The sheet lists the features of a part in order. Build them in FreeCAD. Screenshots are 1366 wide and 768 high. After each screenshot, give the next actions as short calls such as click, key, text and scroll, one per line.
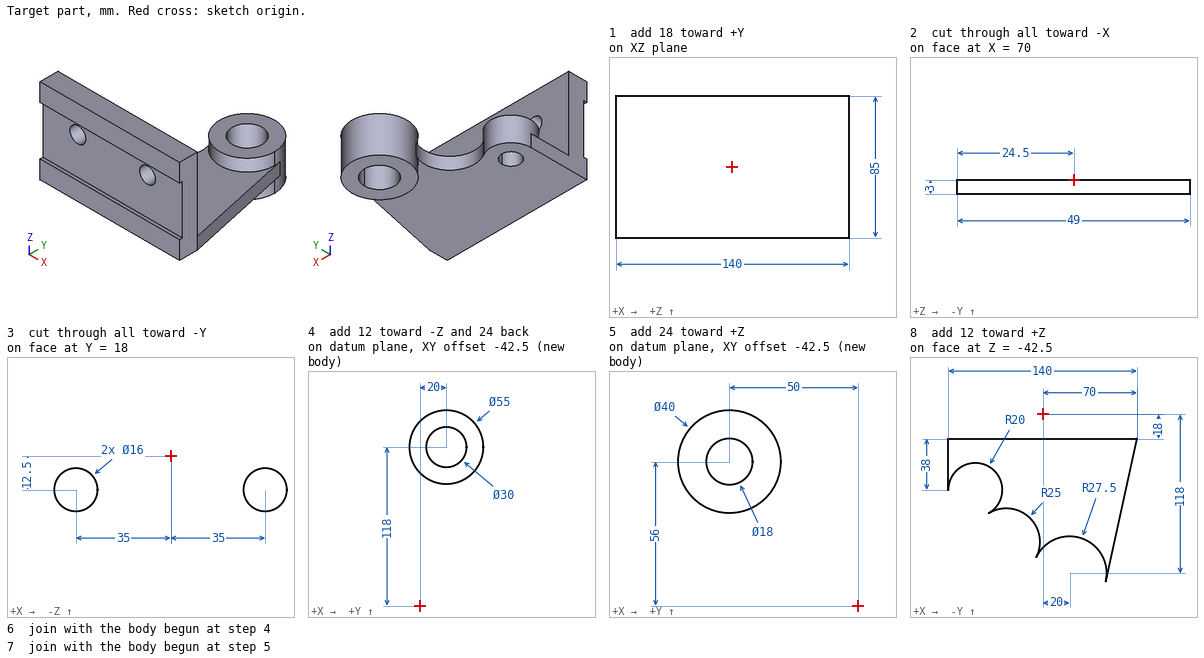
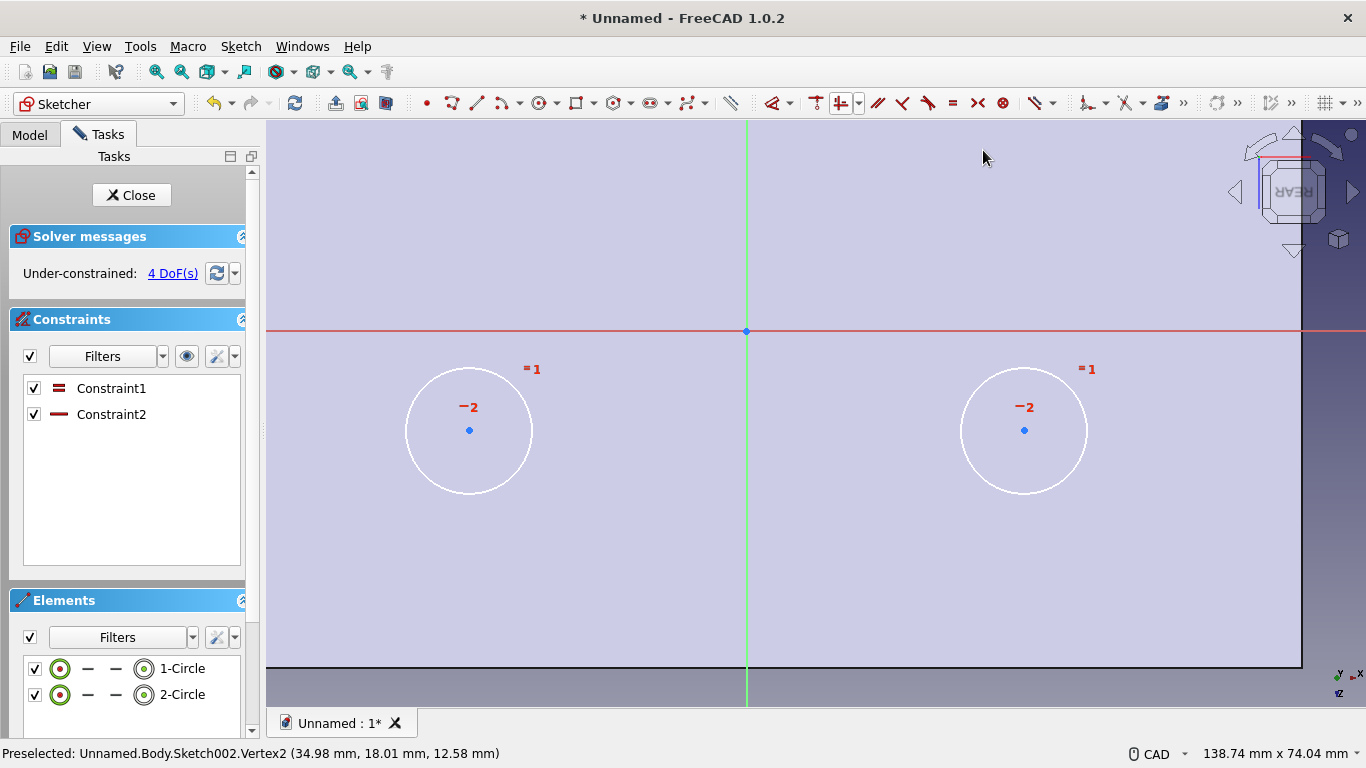
click(772, 104)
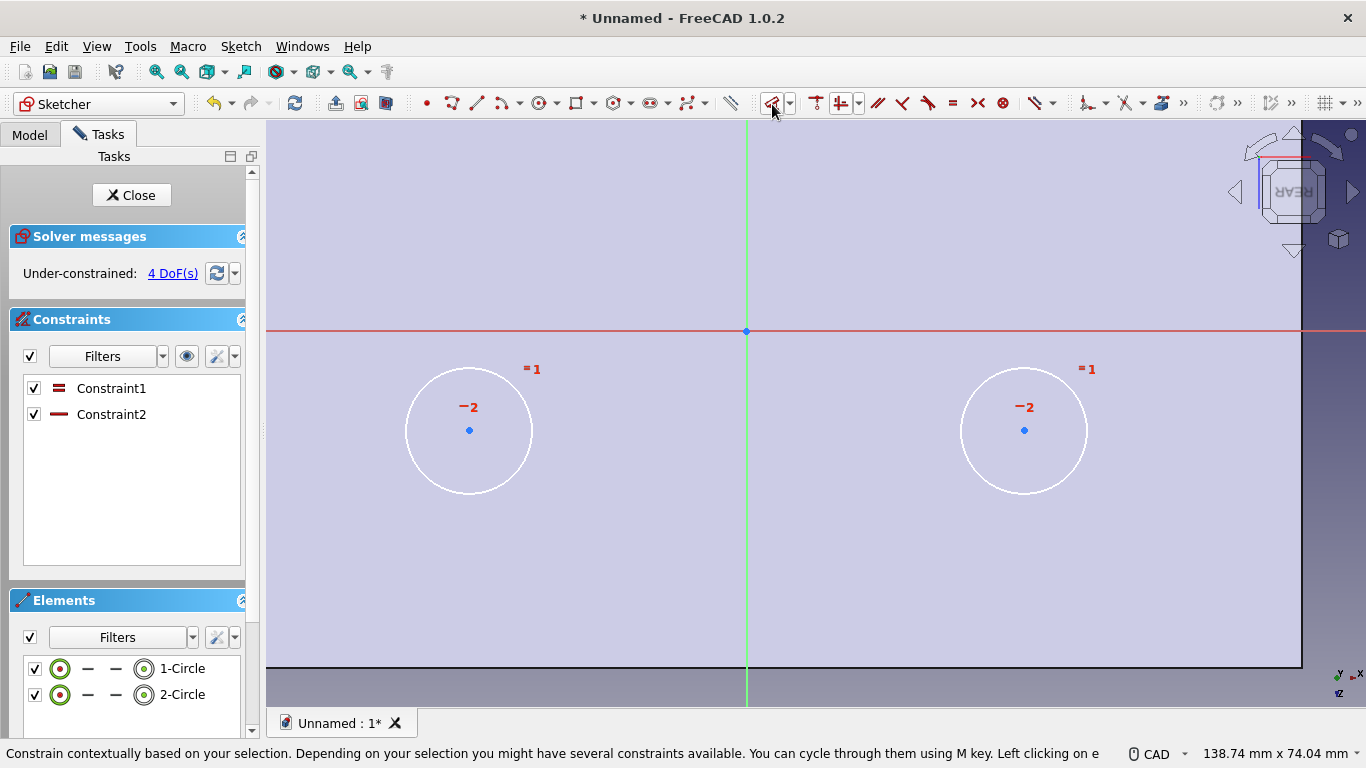
click(513, 386)
click(535, 363)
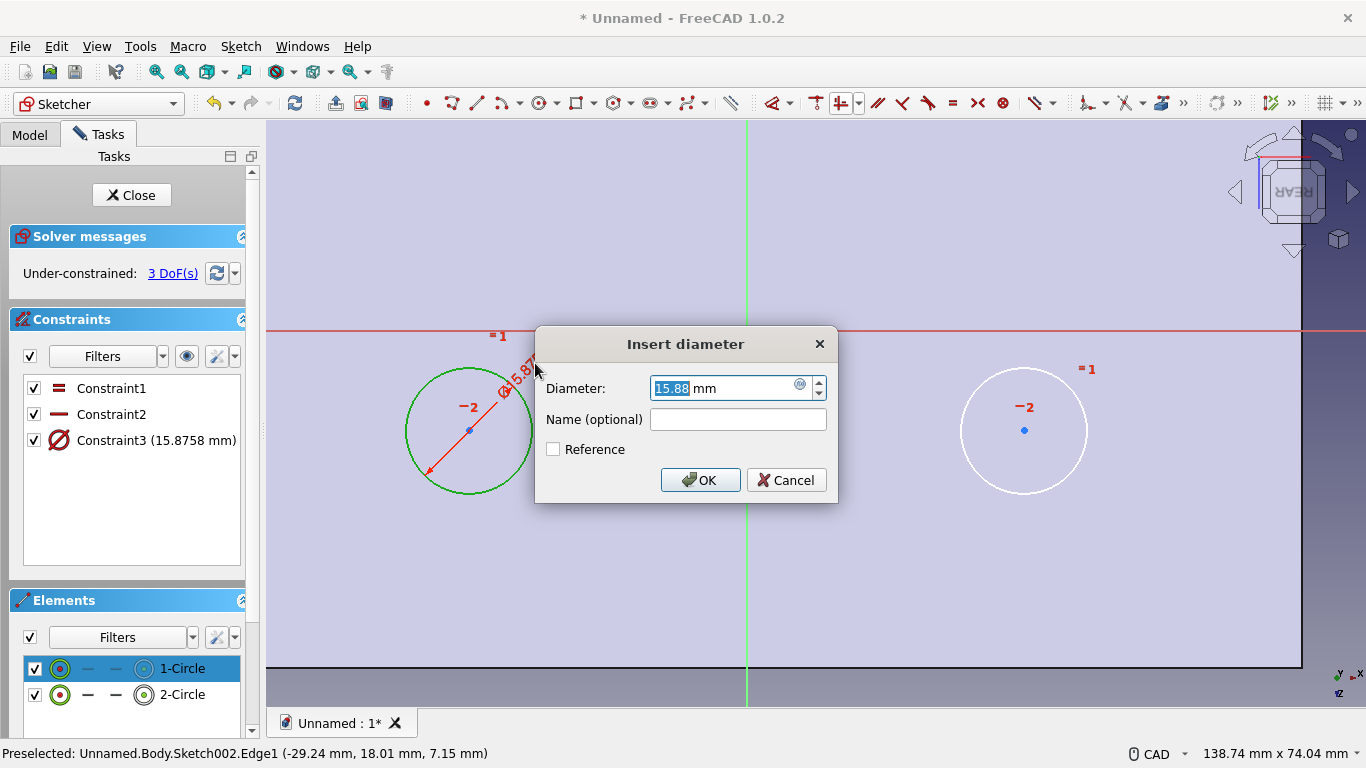
text(16)
key(Return)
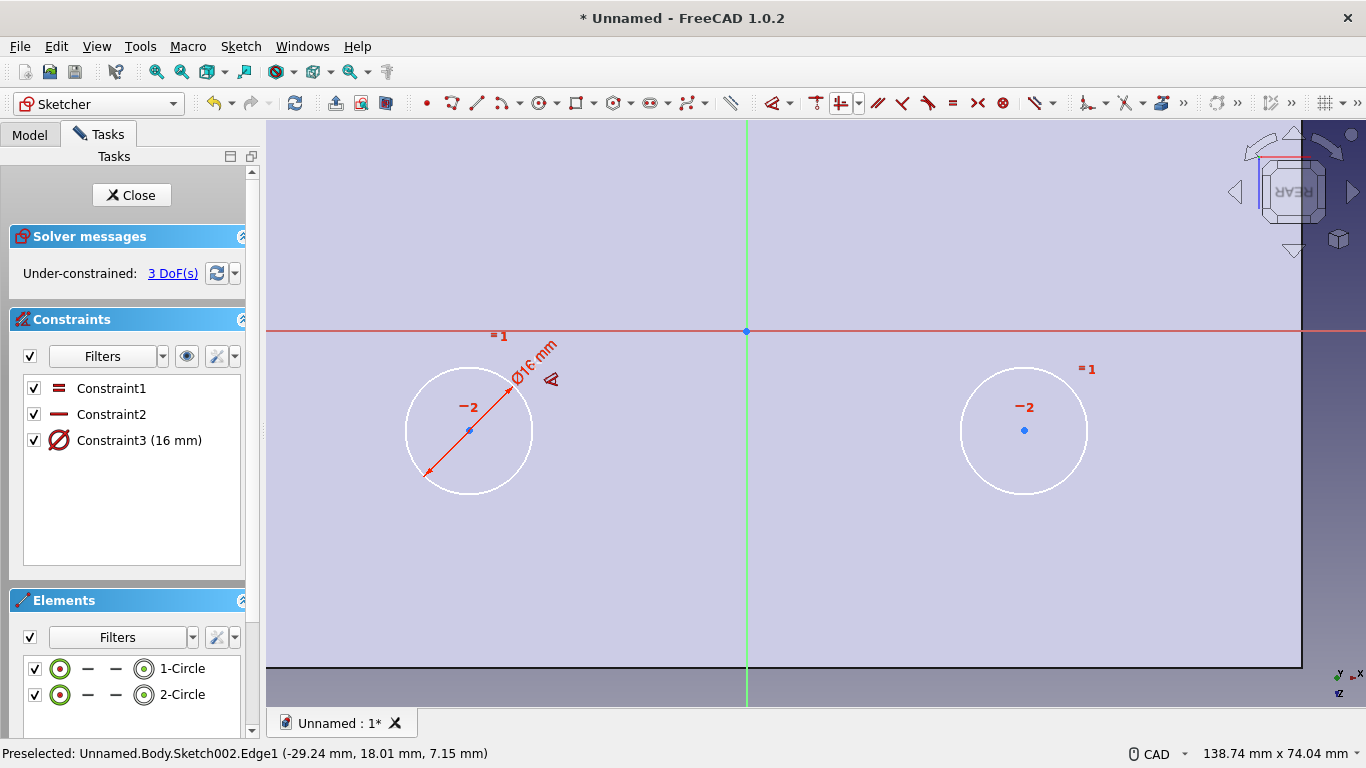
click(469, 431)
click(608, 297)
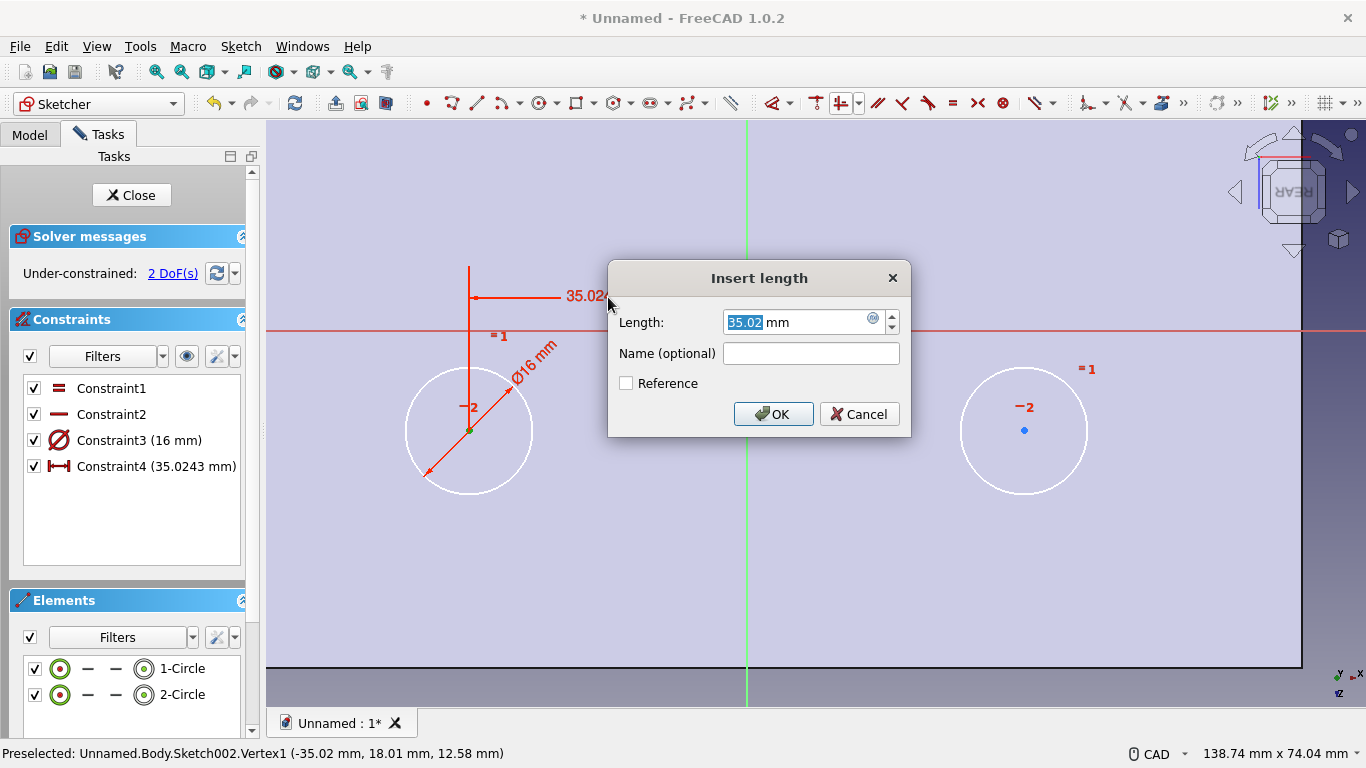
text(35)
key(Return)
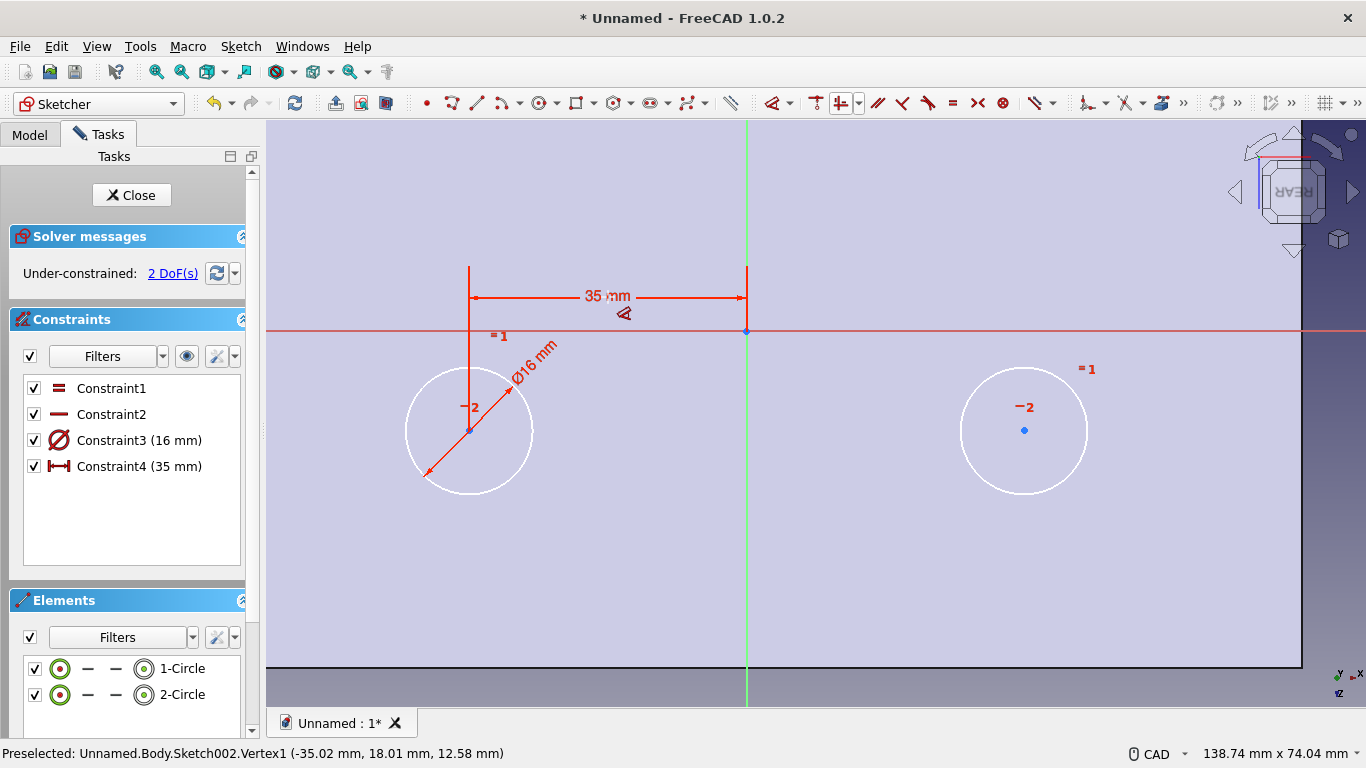
click(1024, 431)
click(885, 297)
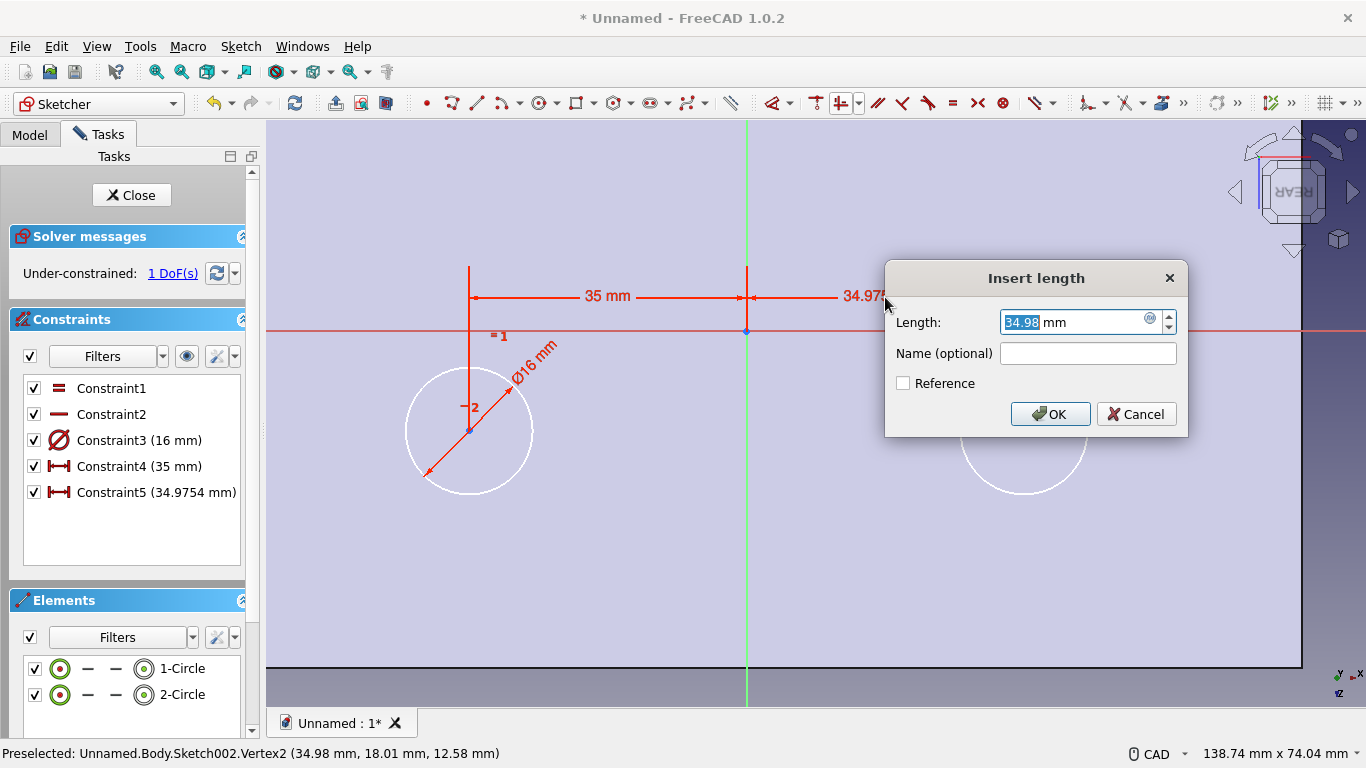
text(35)
key(Return)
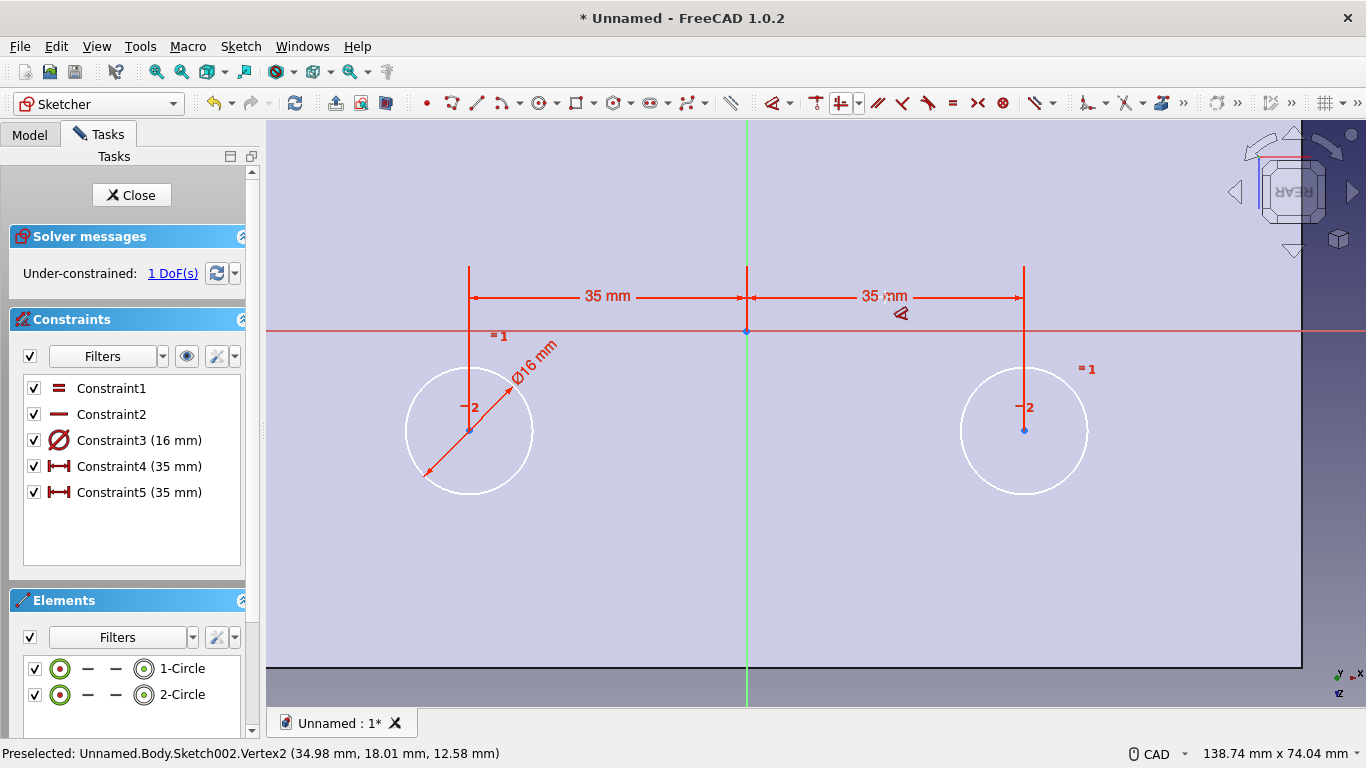
click(469, 431)
click(435, 358)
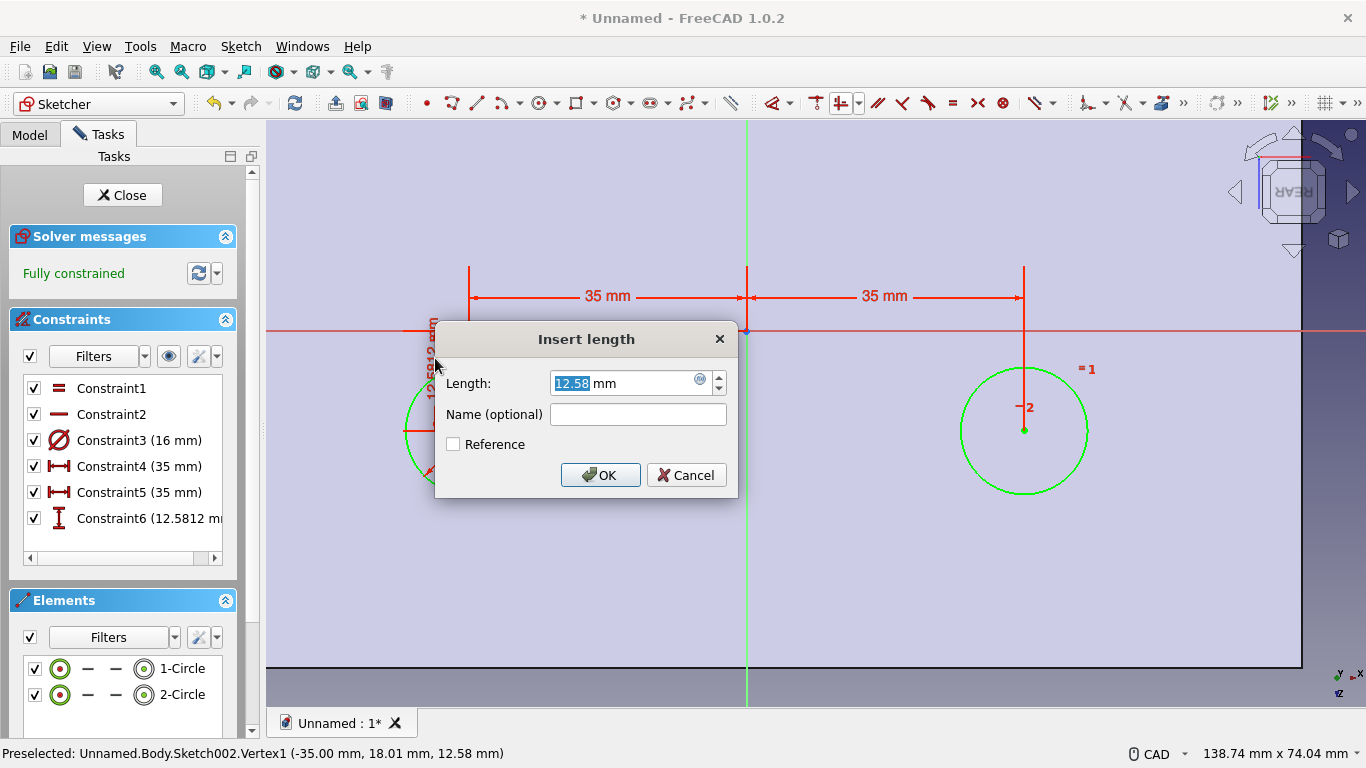
text(12.5)
key(Return)
key(Escape)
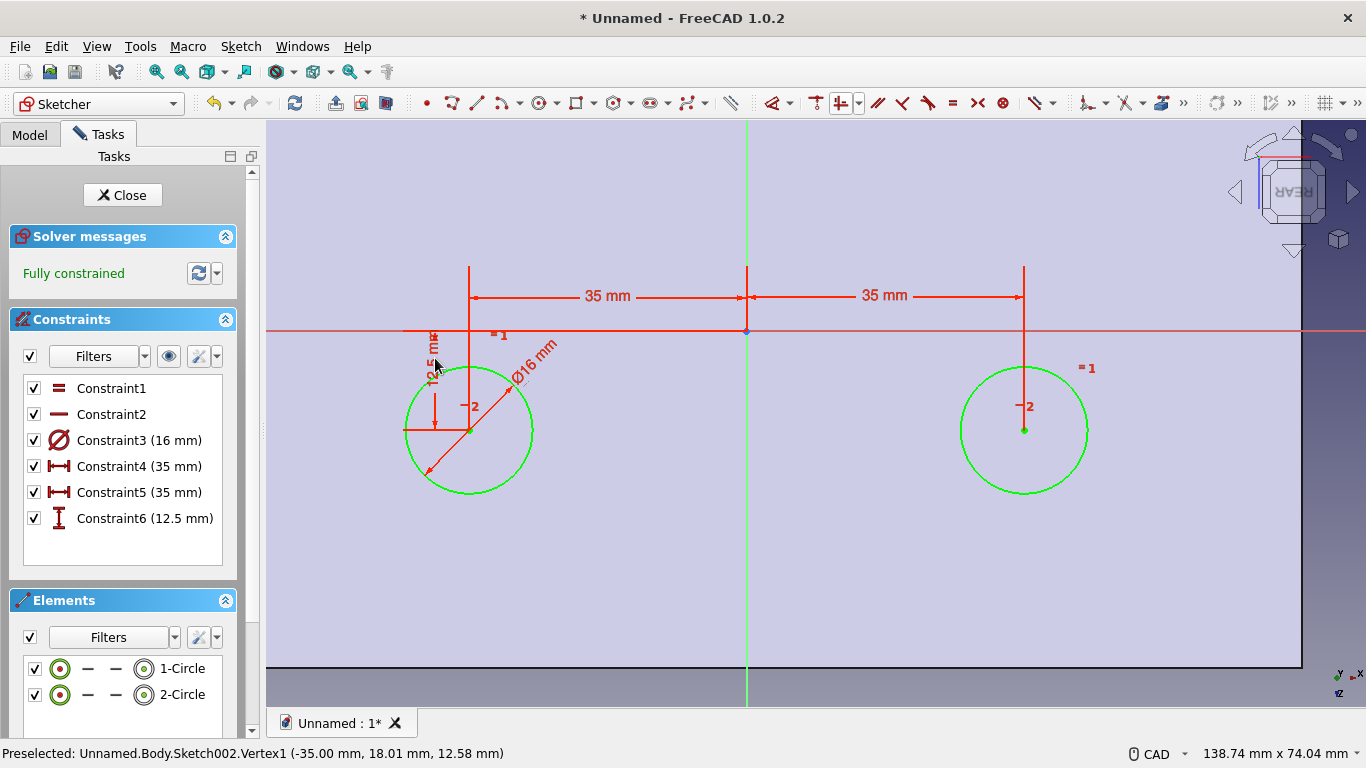
click(123, 195)